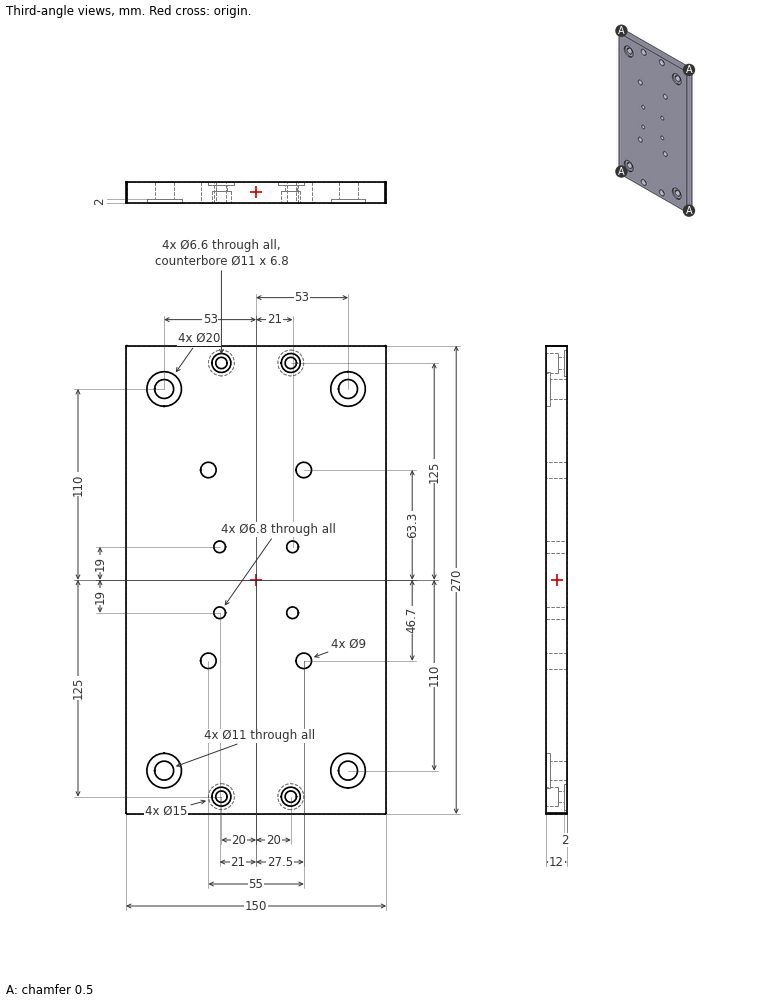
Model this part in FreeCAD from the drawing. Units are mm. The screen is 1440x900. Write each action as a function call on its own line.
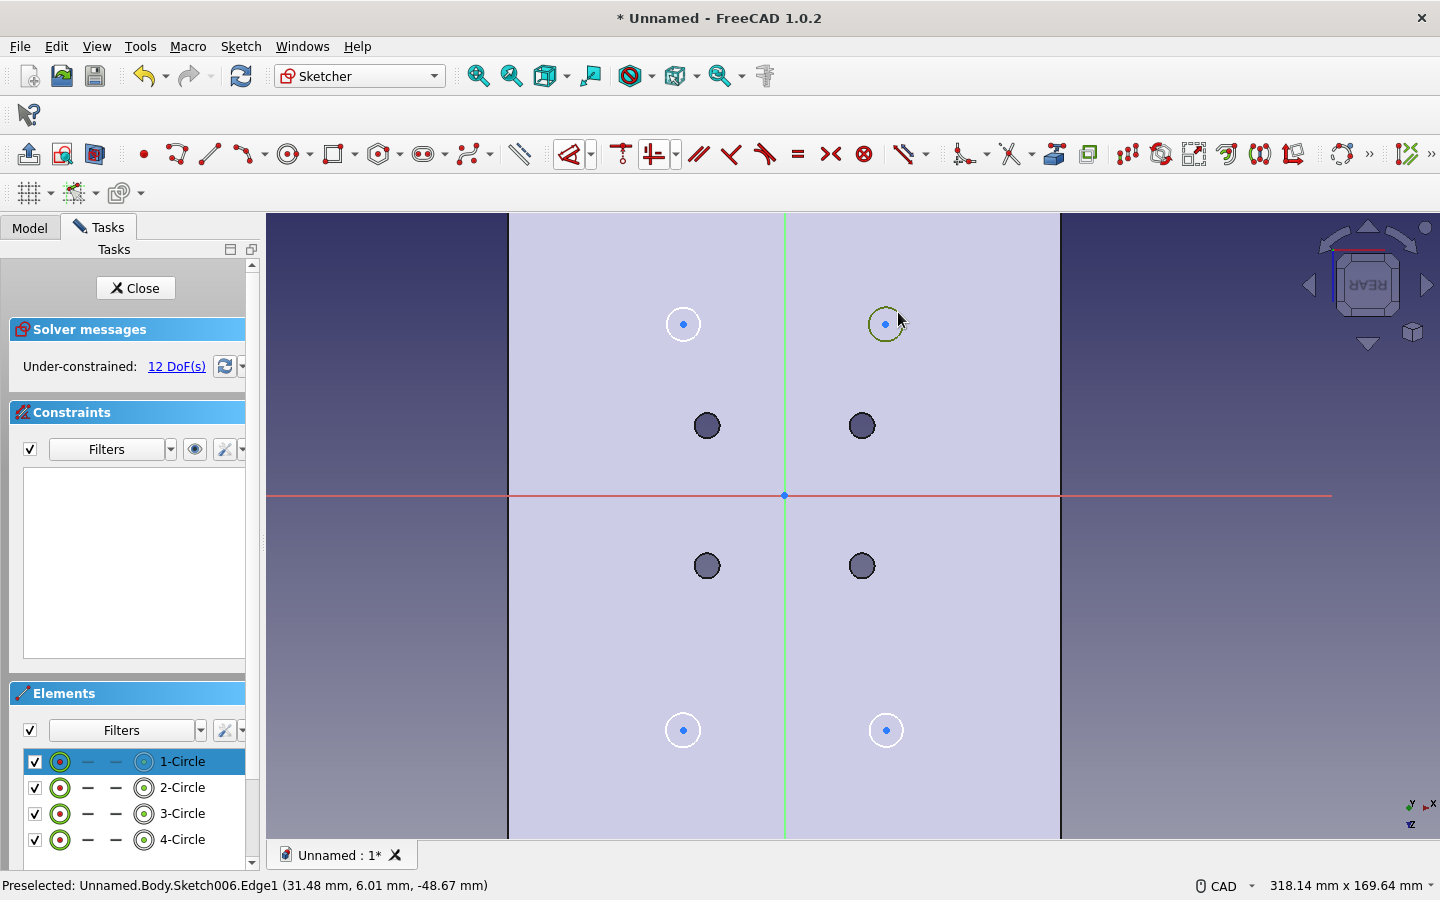
click(695, 313)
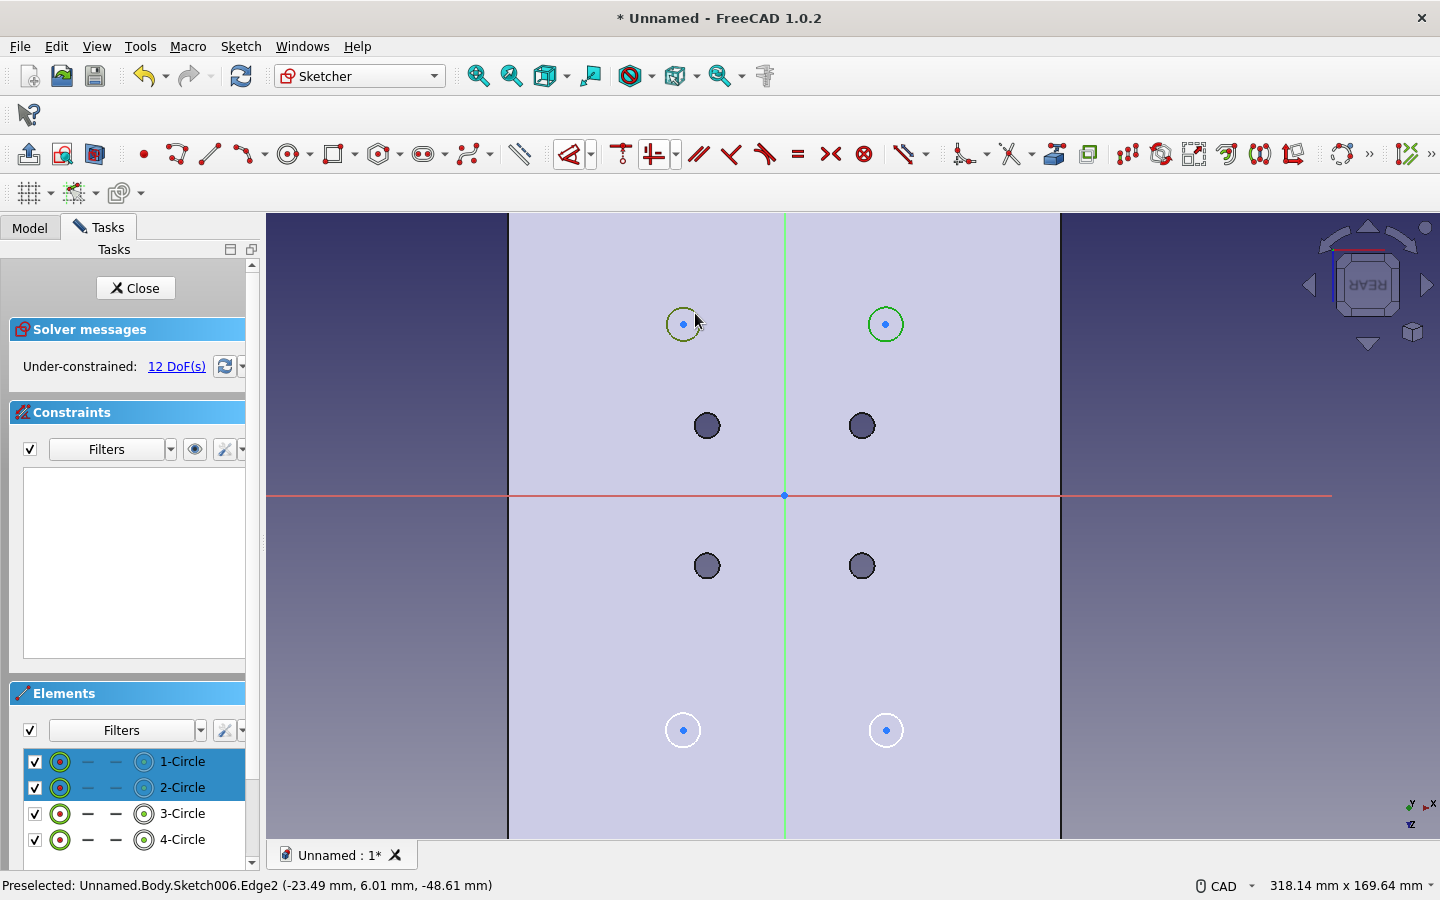
click(898, 719)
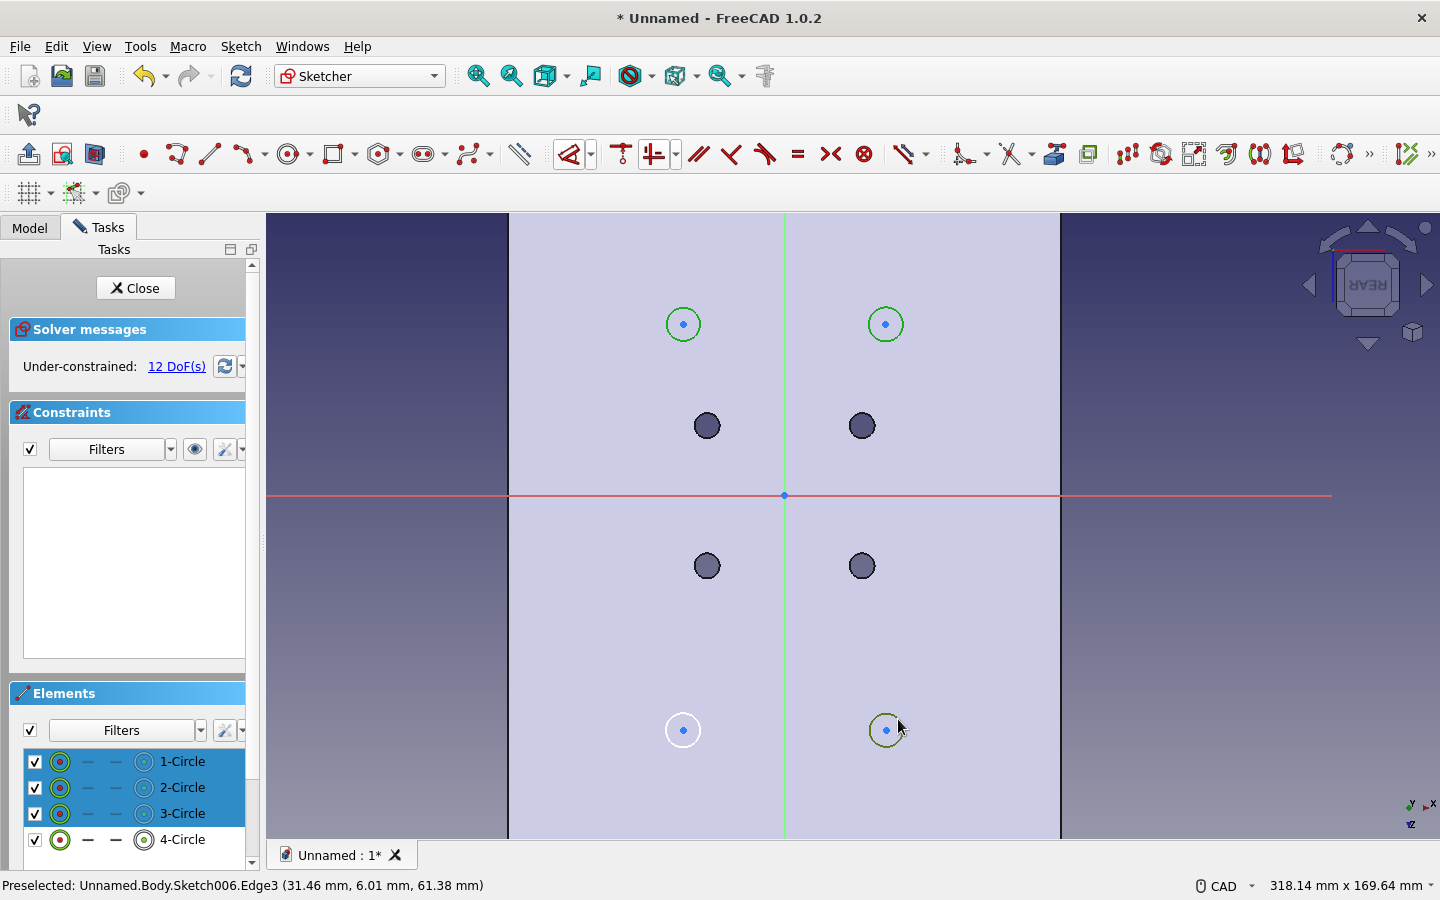
click(695, 718)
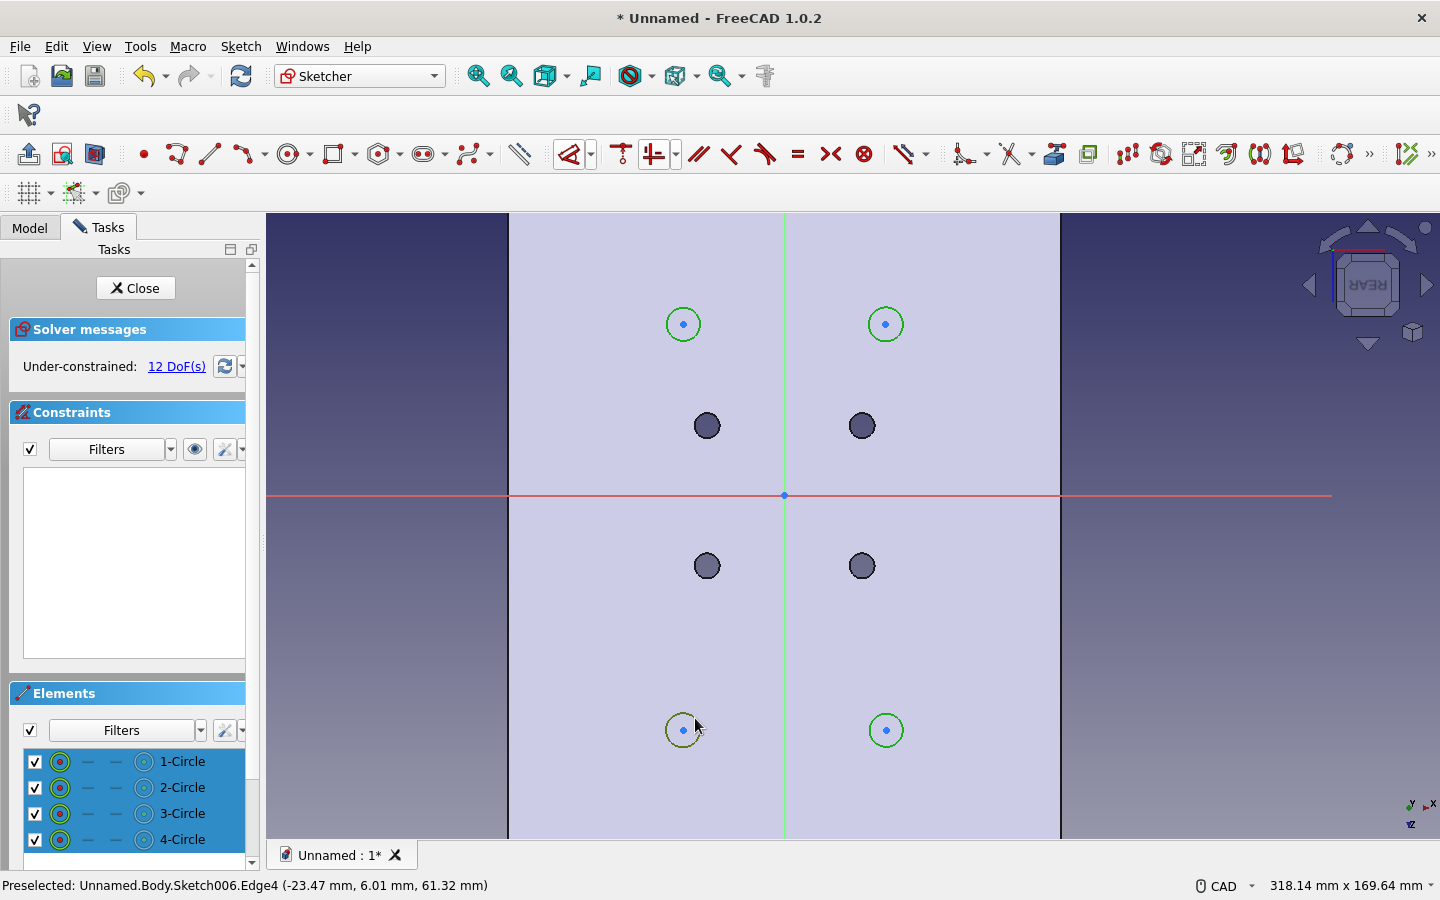
key(e)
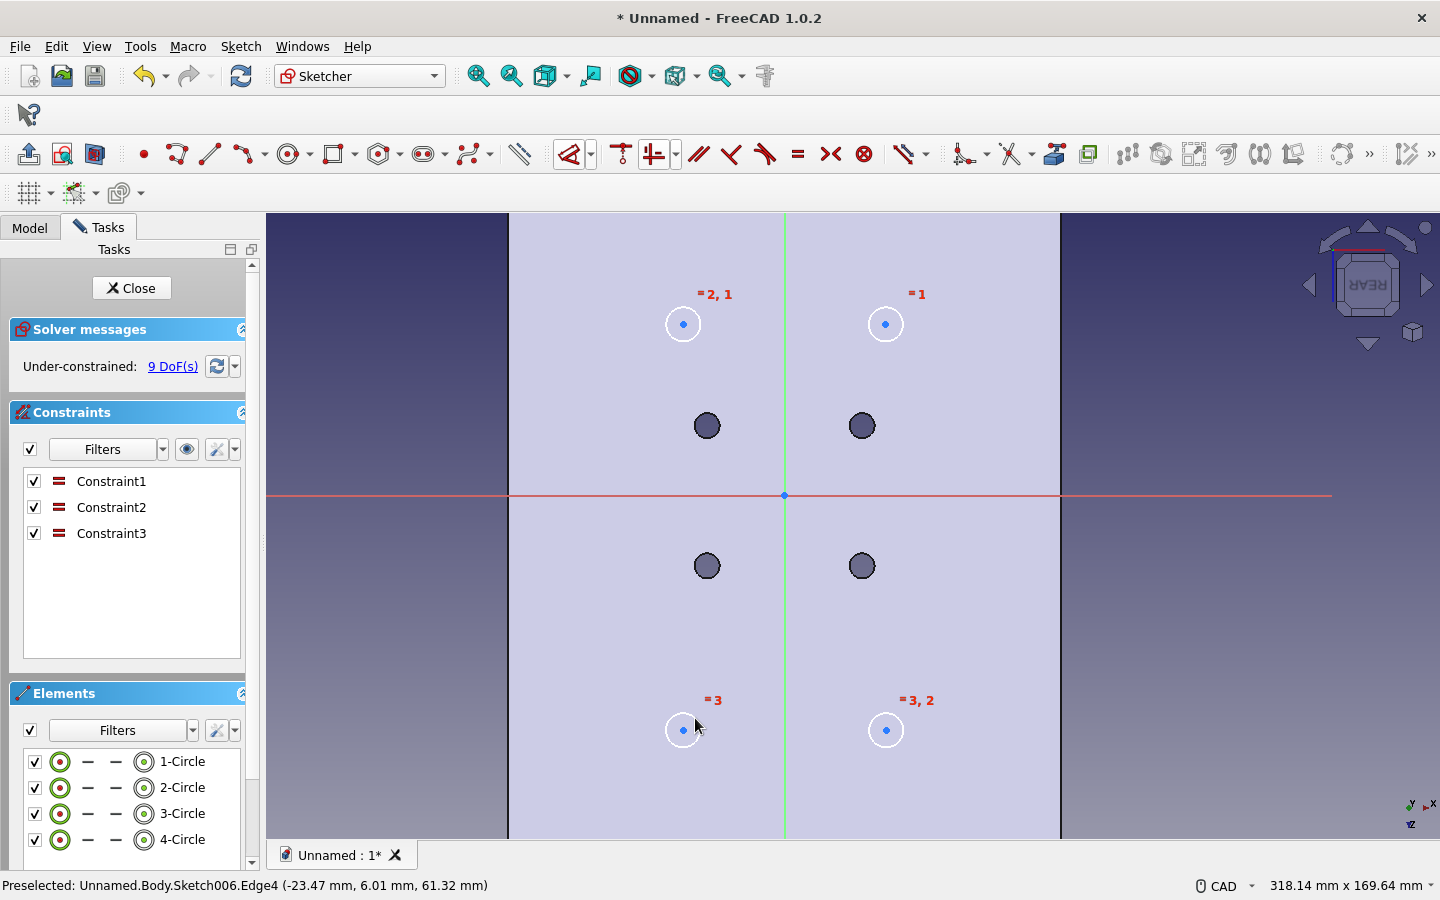
click(886, 324)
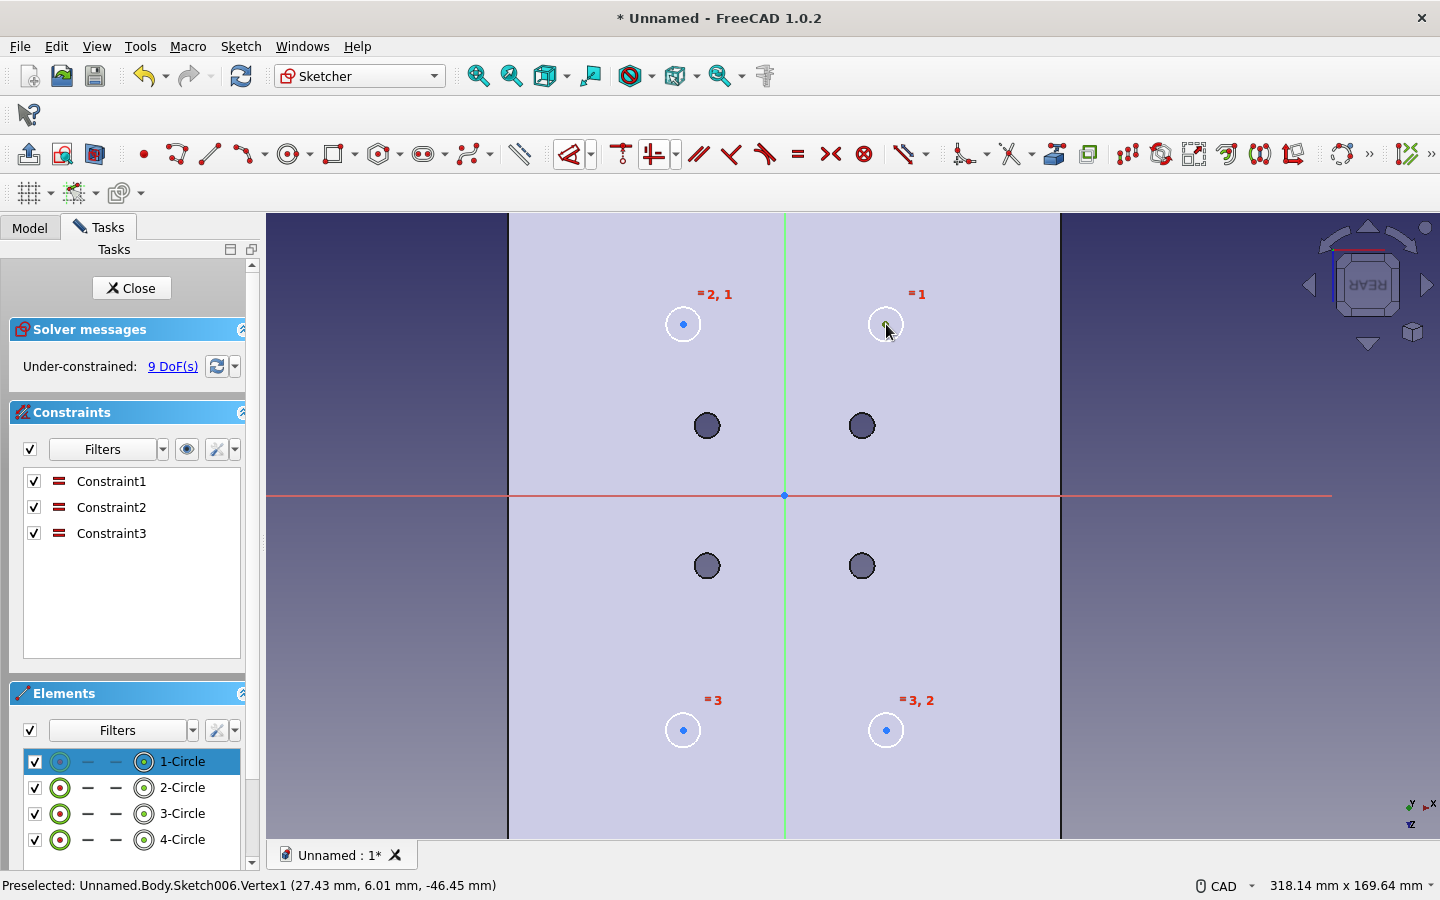
click(683, 324)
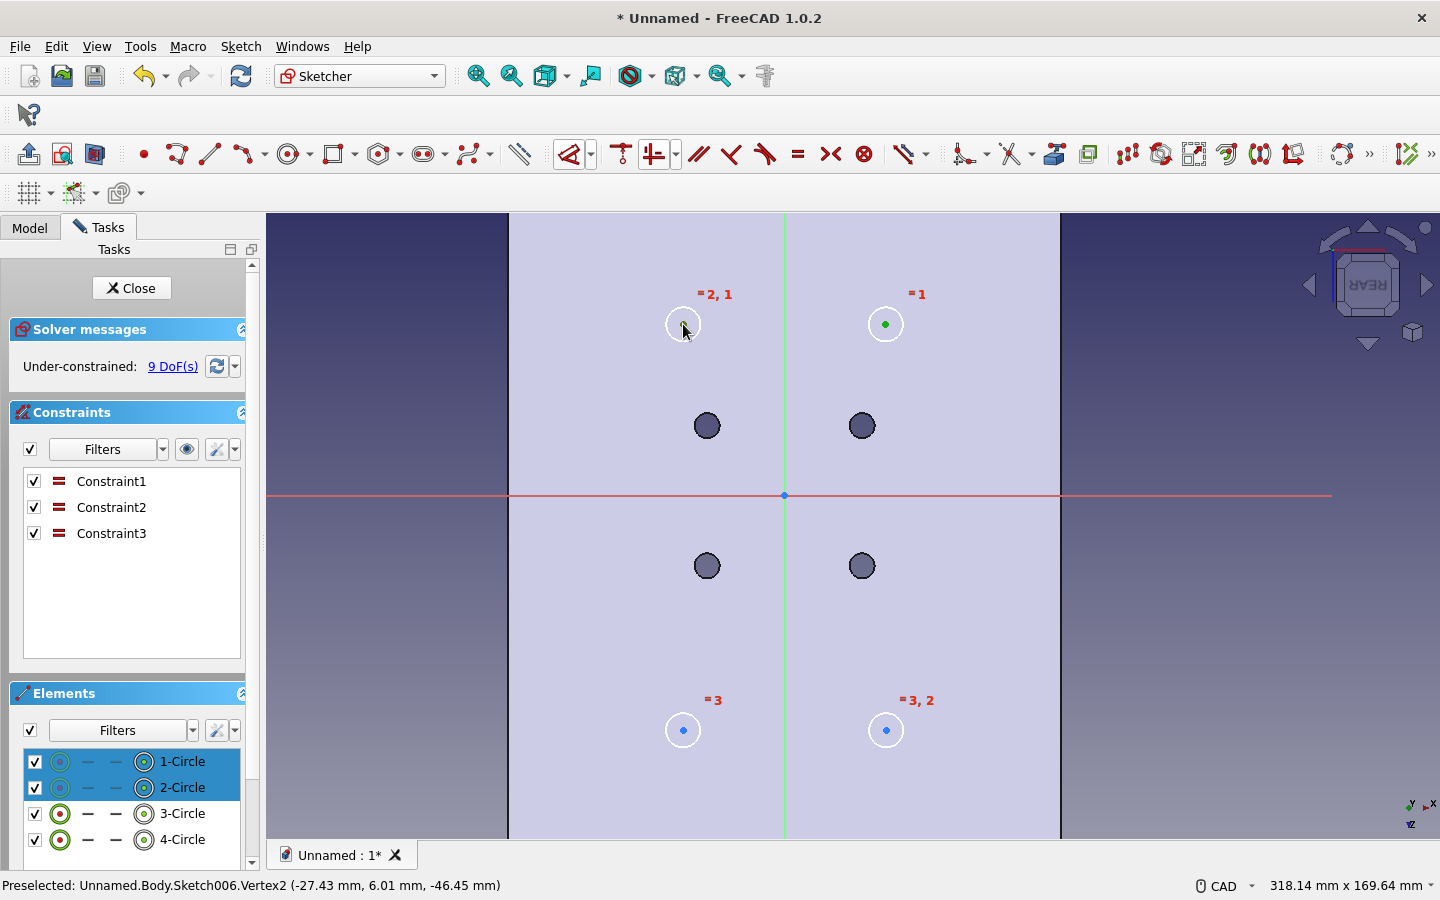
key(h)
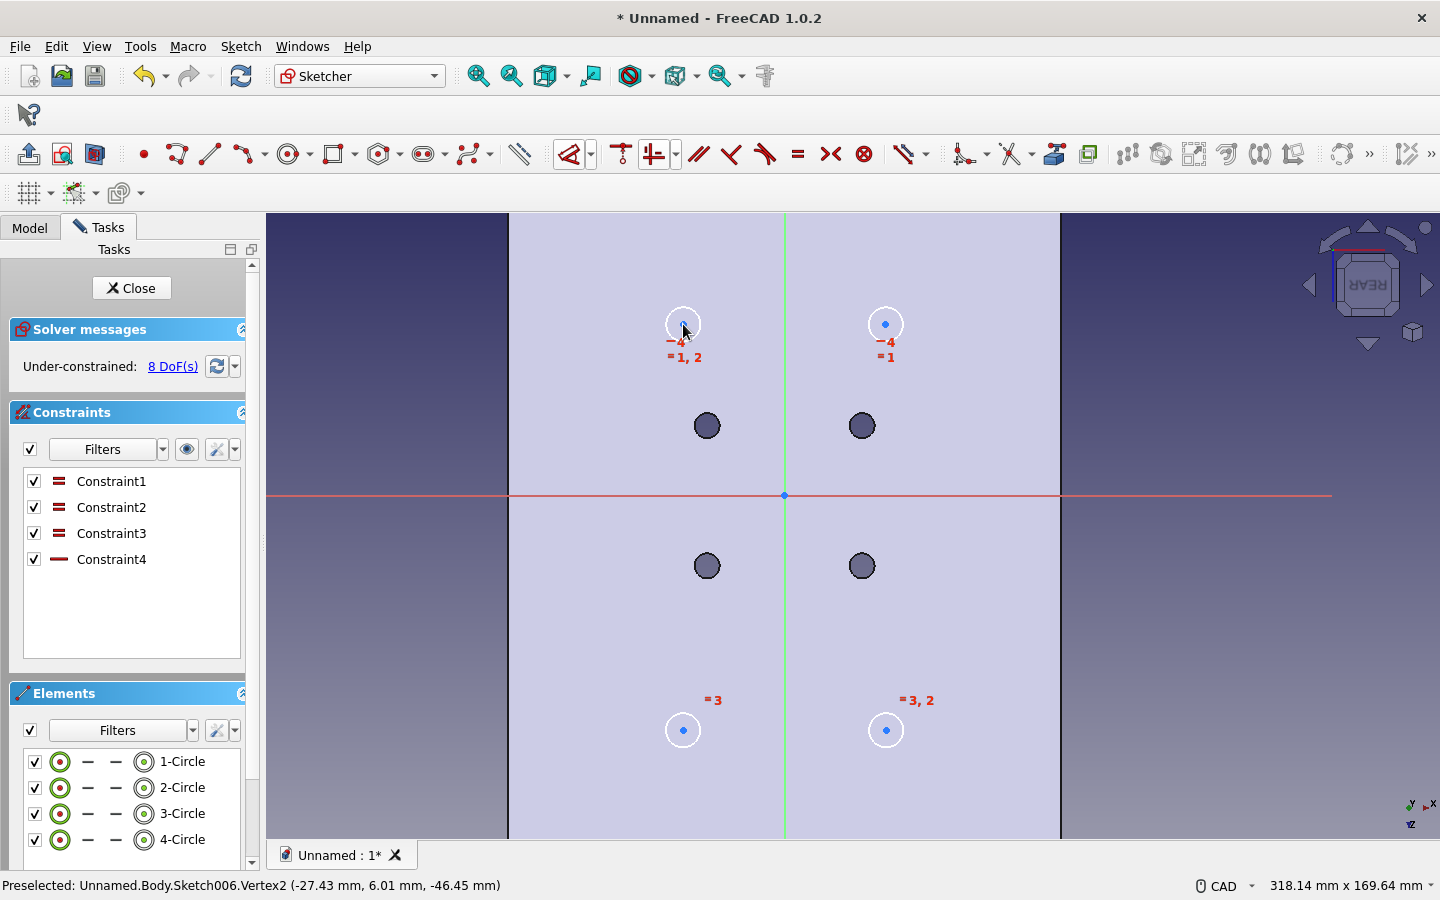
click(886, 324)